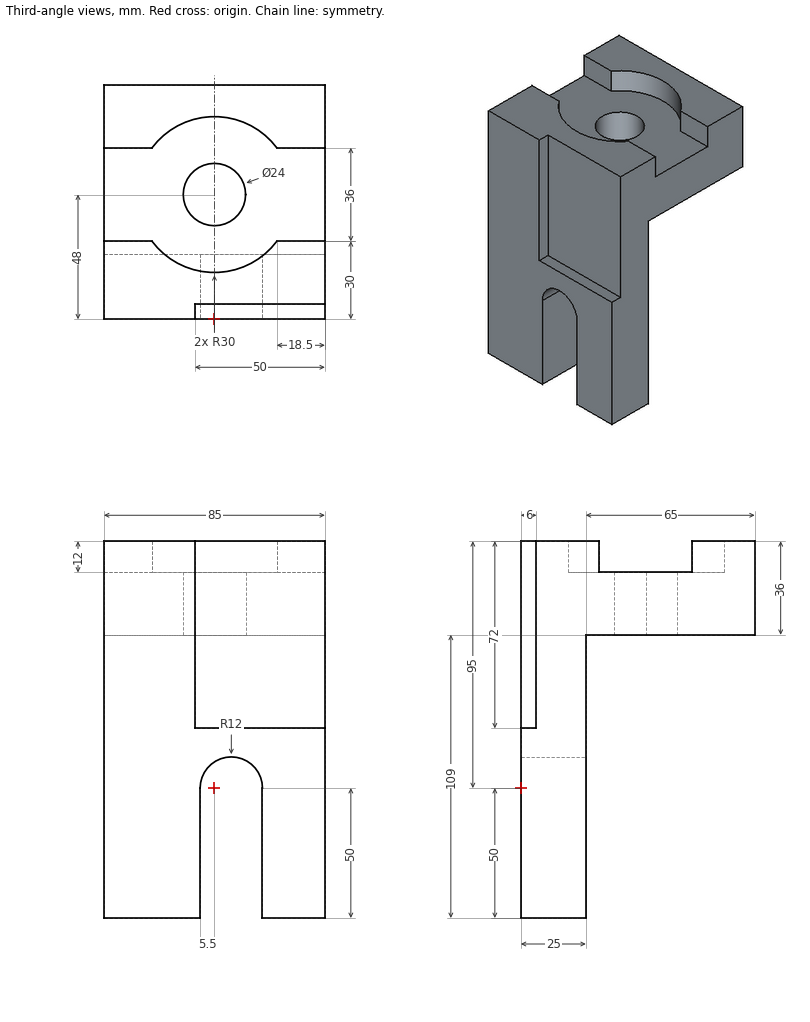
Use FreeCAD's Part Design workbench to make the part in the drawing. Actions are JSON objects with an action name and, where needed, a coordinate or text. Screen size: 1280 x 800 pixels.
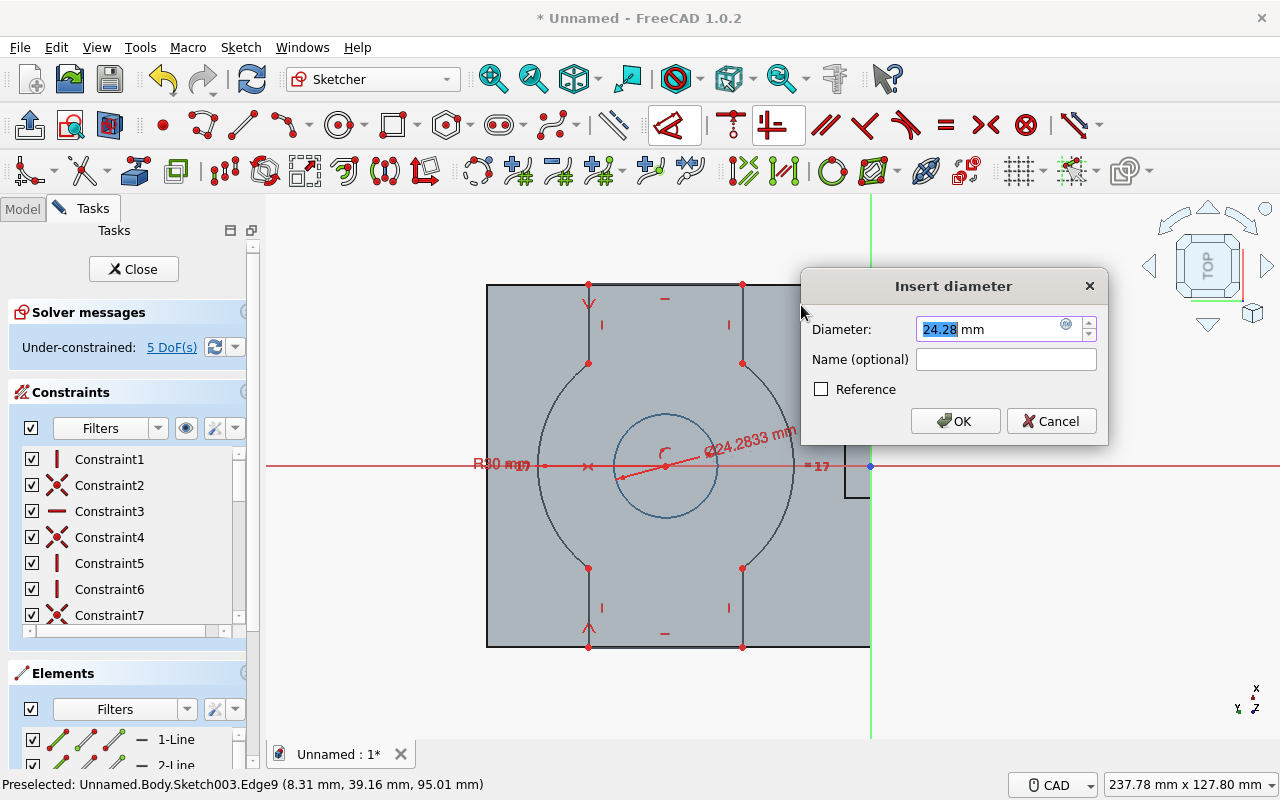
{"action": "type", "text": "24"}
{"action": "key", "text": "Return"}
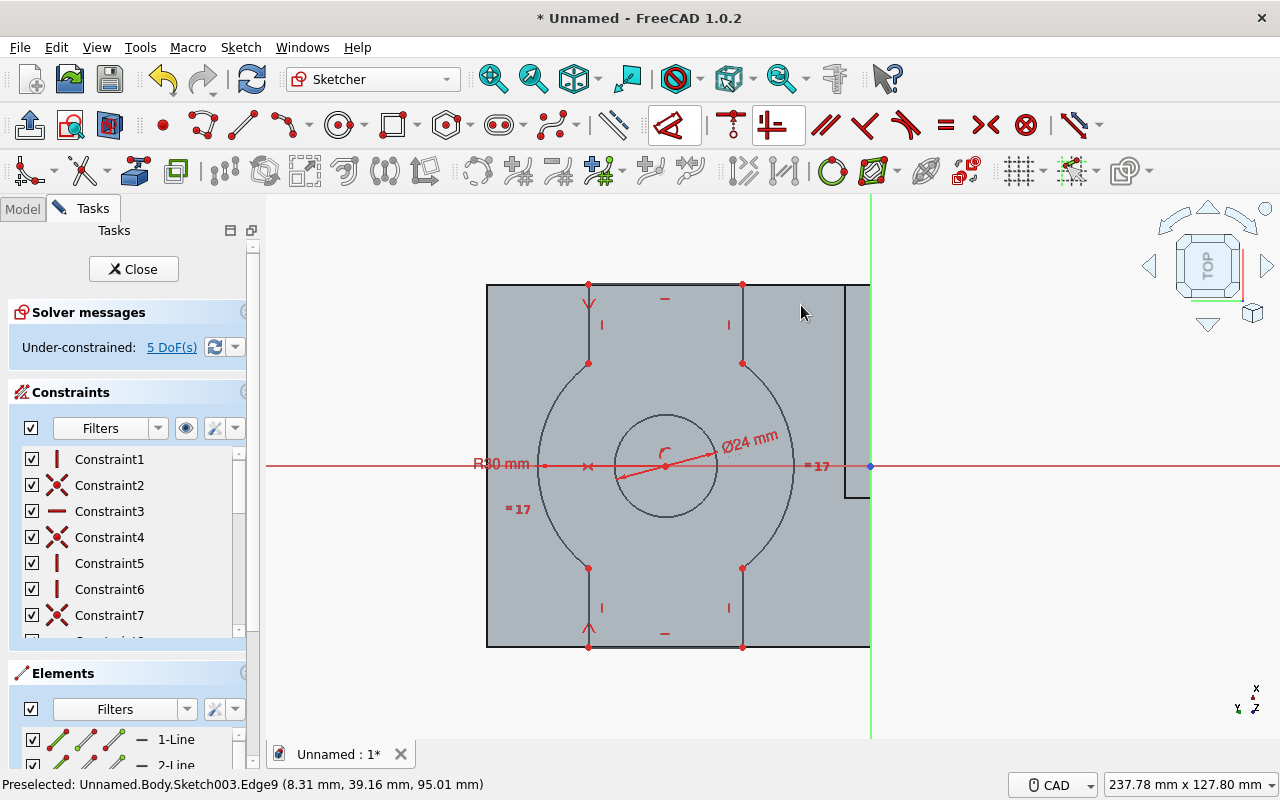
{"action": "left_click", "coordinate": [697, 284]}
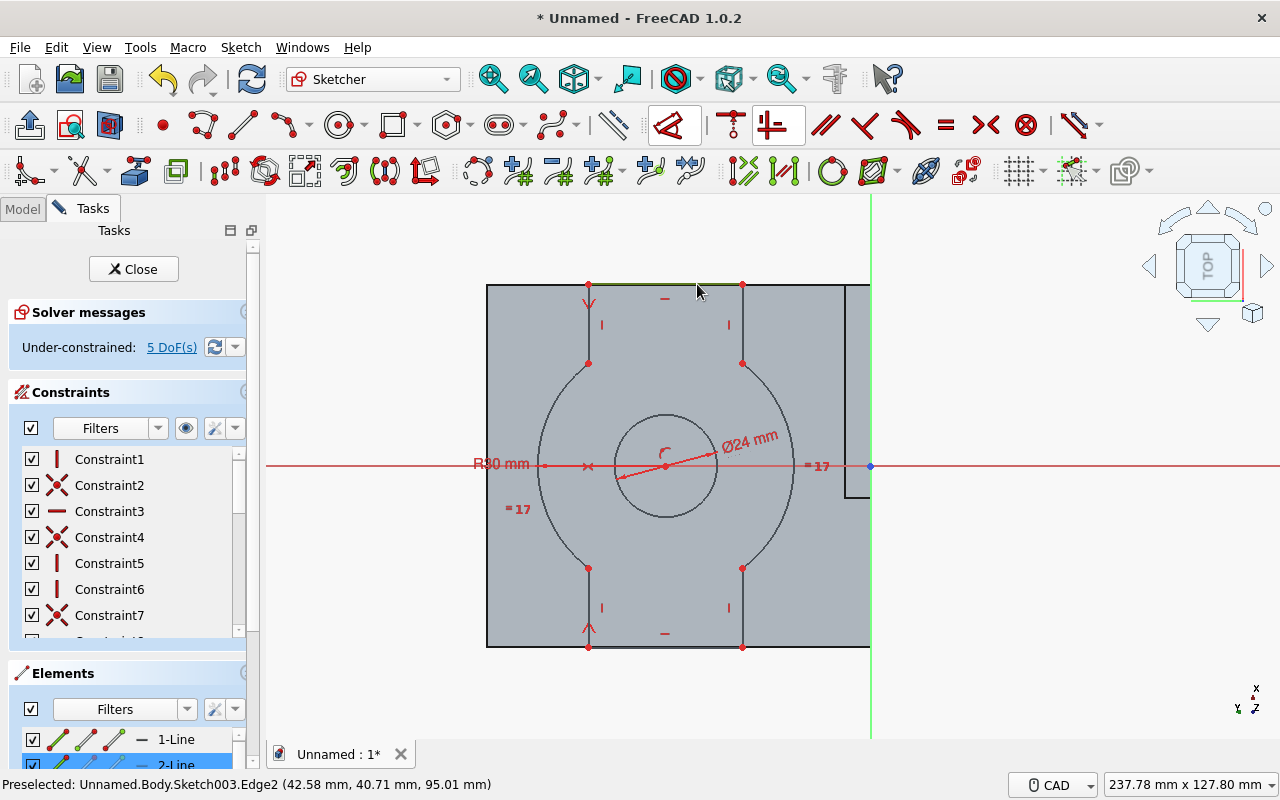
{"action": "left_click", "coordinate": [696, 126]}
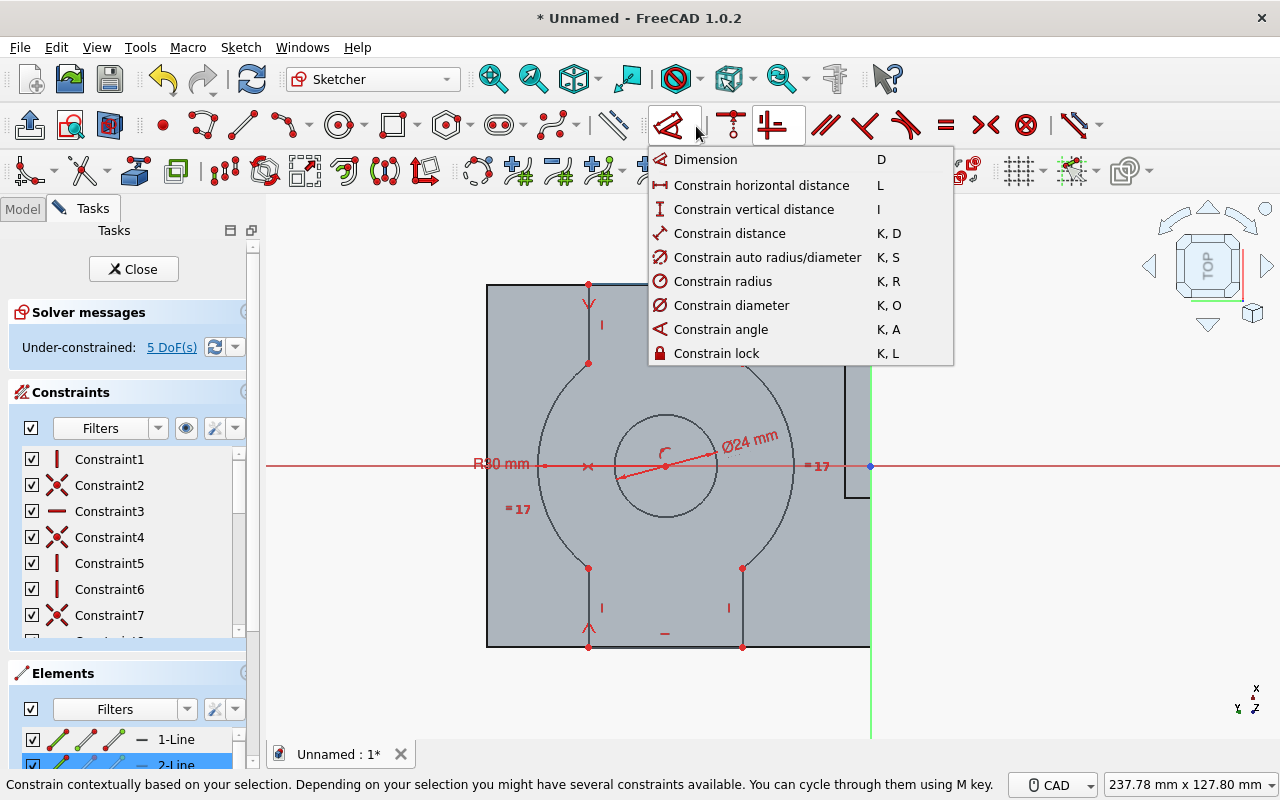
{"action": "left_click", "coordinate": [801, 185]}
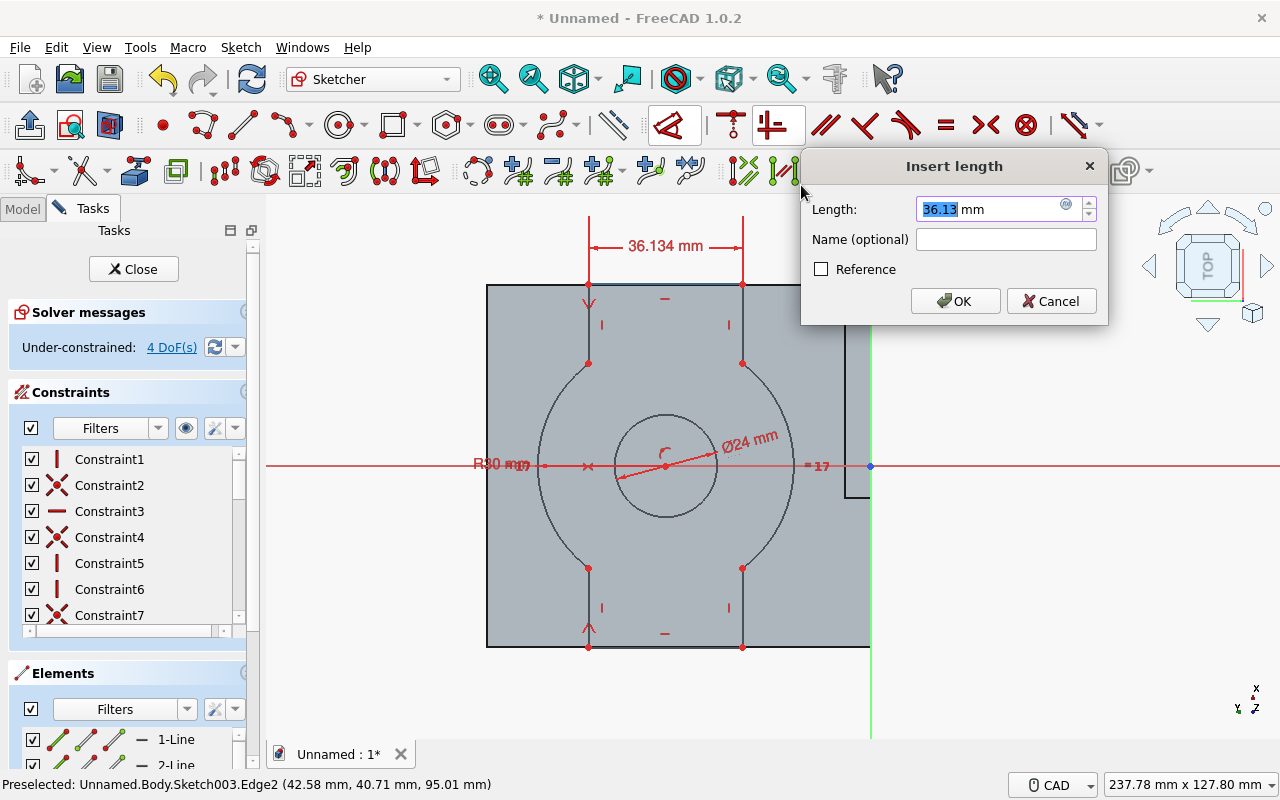
{"action": "type", "text": "36"}
{"action": "key", "text": "Return"}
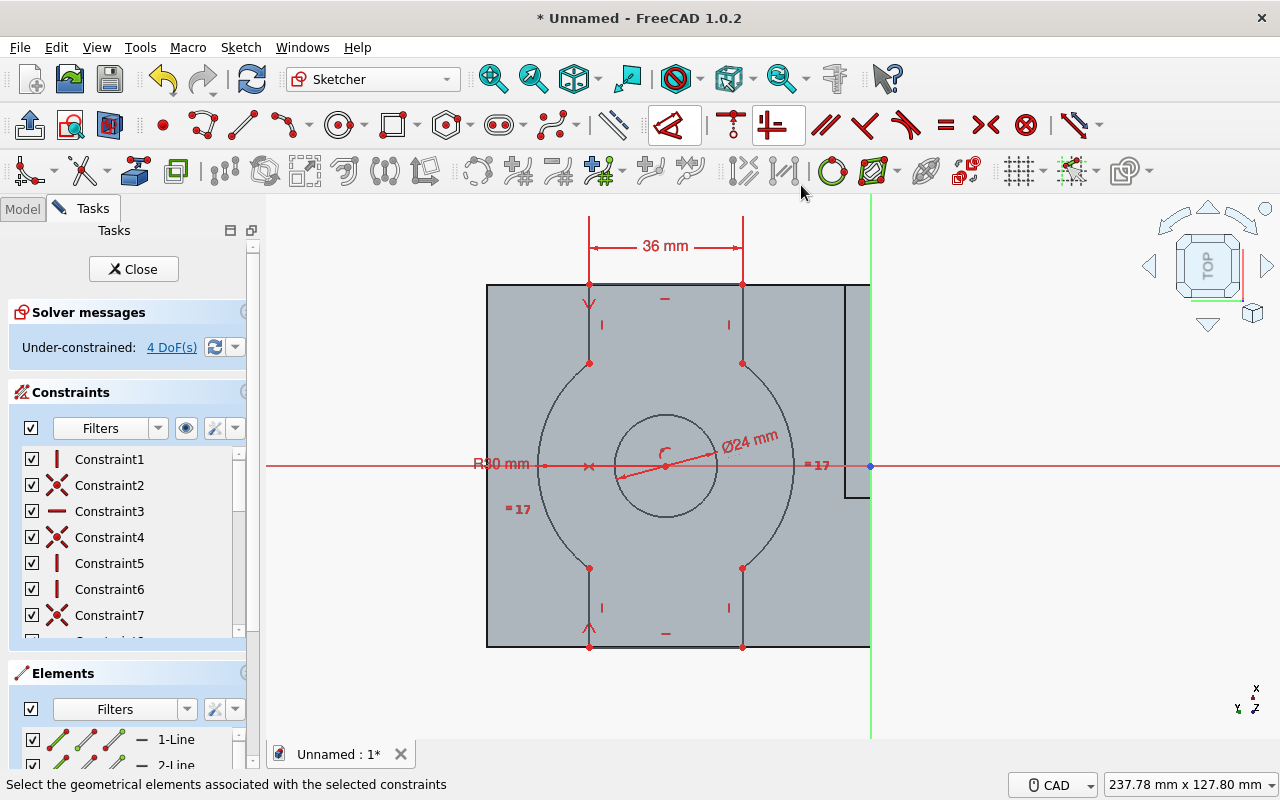
{"action": "left_click", "coordinate": [635, 648]}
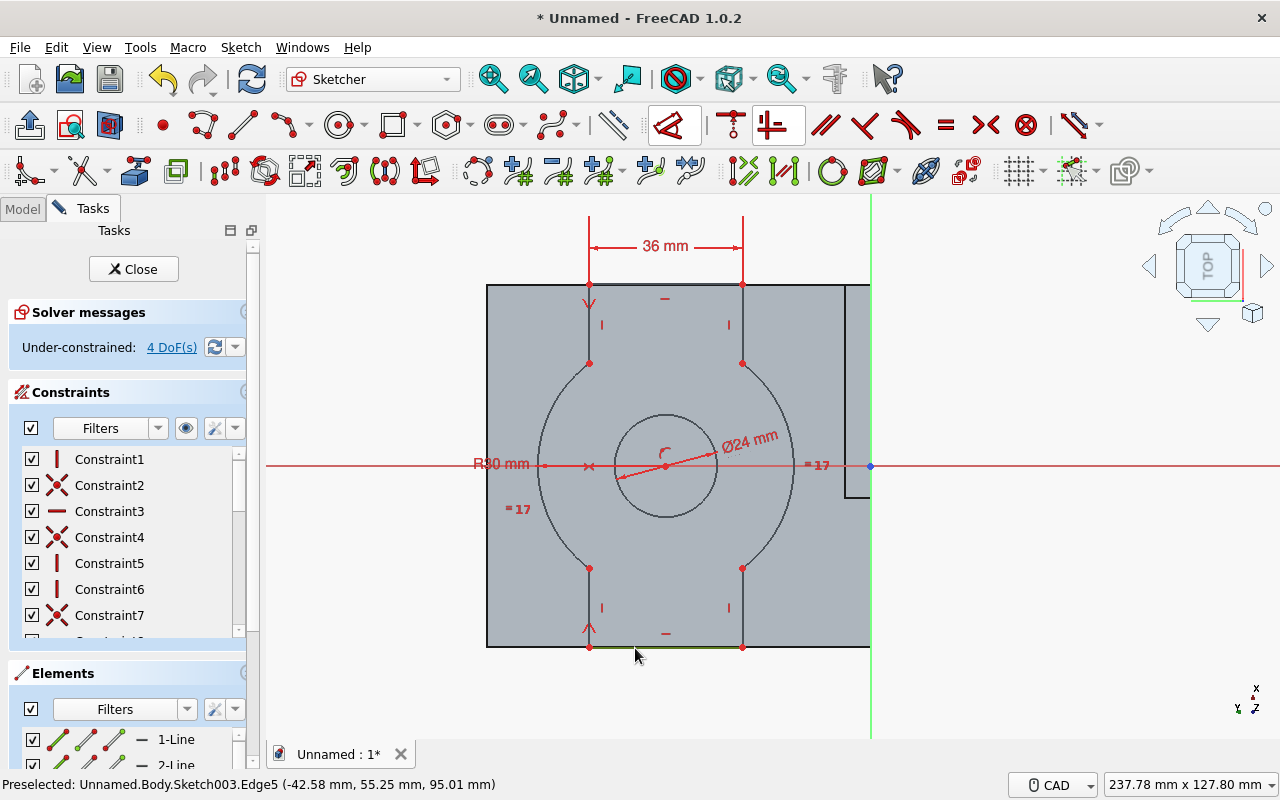
{"action": "left_click", "coordinate": [696, 126]}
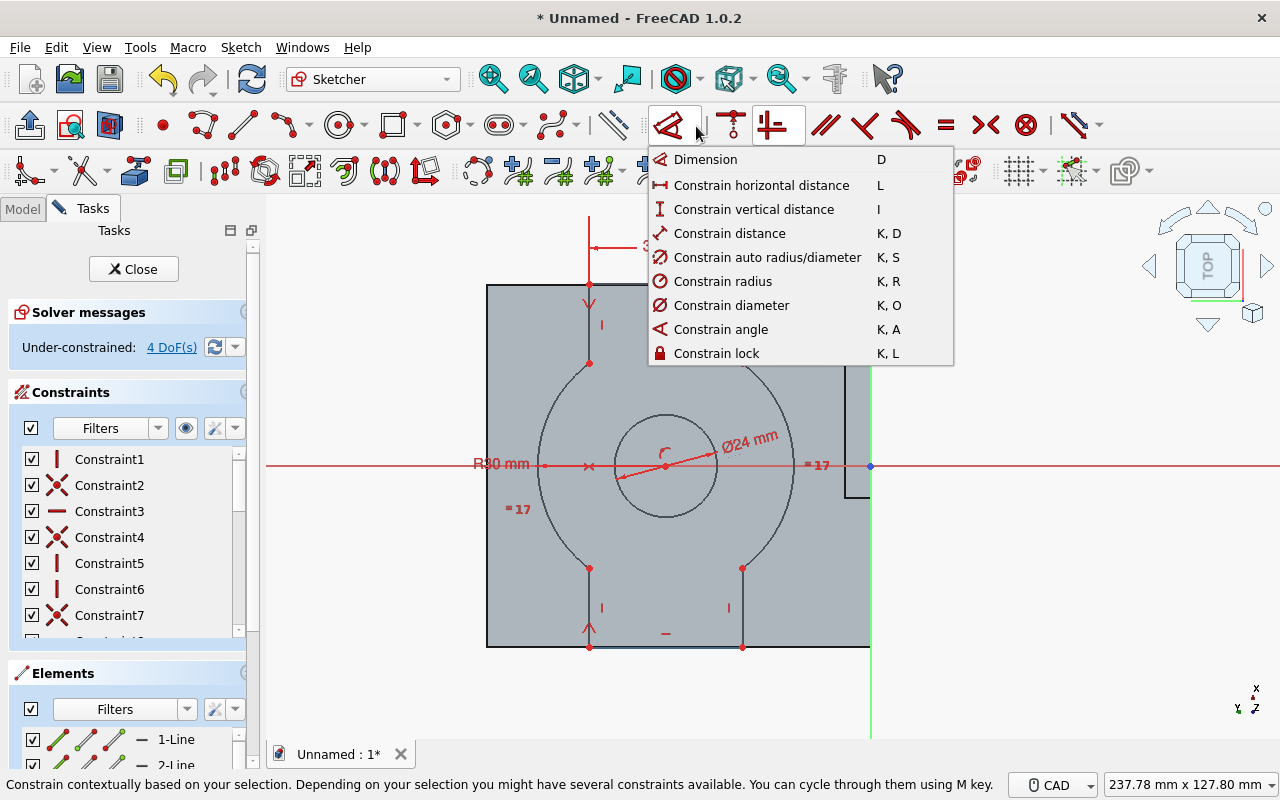
{"action": "left_click", "coordinate": [801, 185]}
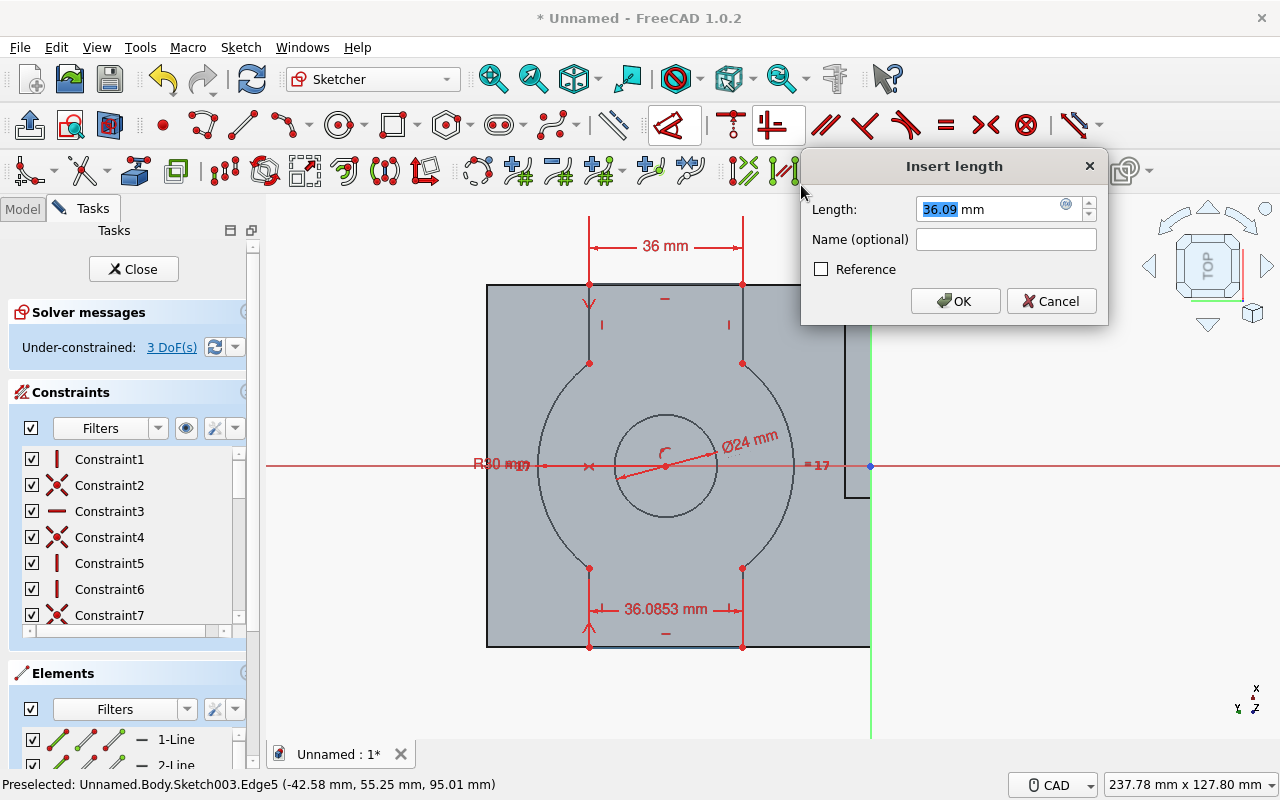
{"action": "type", "text": "36"}
{"action": "key", "text": "Return"}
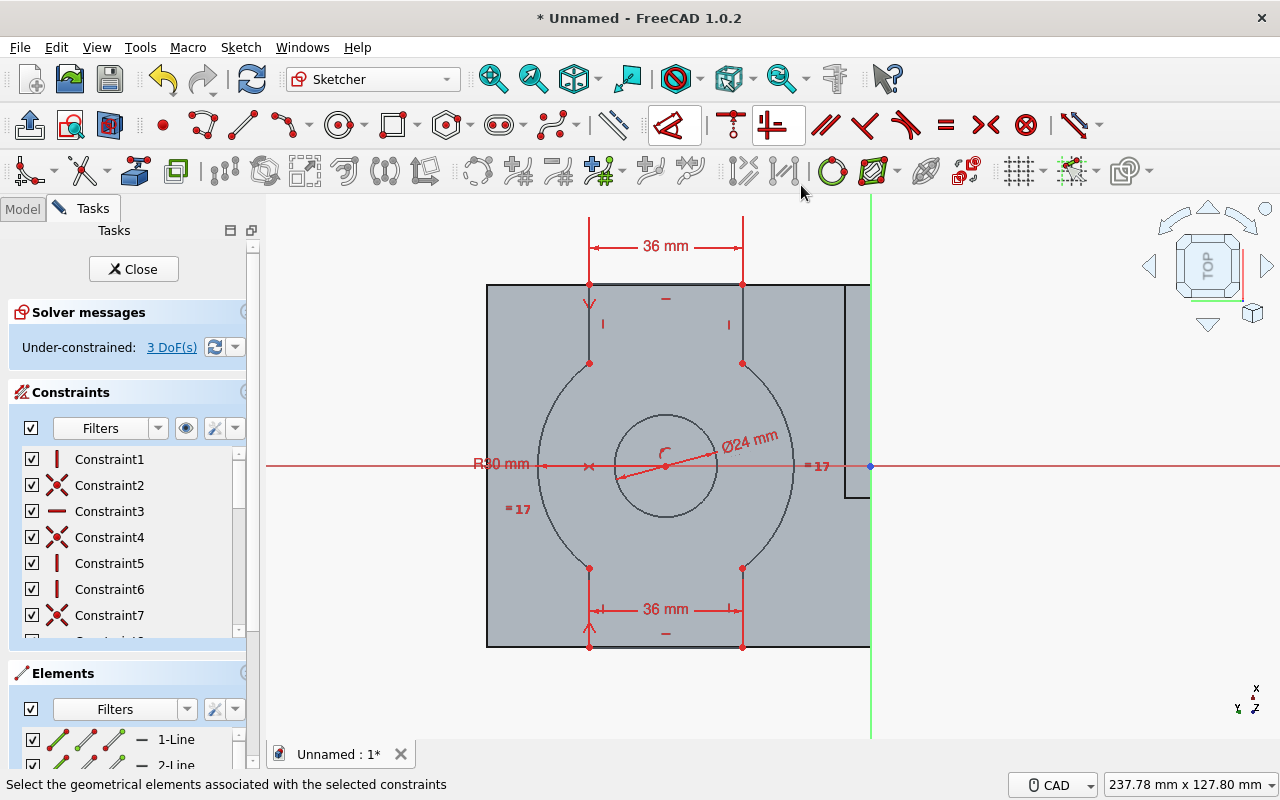
{"action": "left_click", "coordinate": [666, 466]}